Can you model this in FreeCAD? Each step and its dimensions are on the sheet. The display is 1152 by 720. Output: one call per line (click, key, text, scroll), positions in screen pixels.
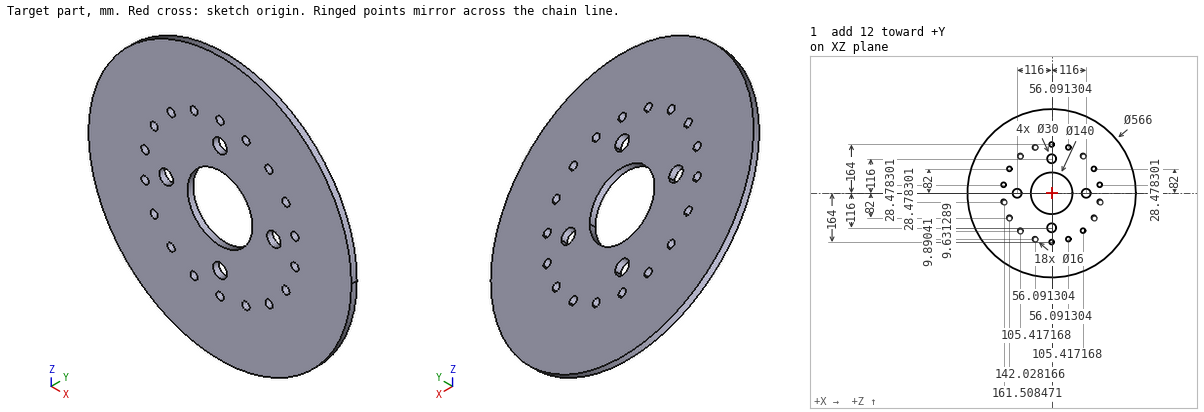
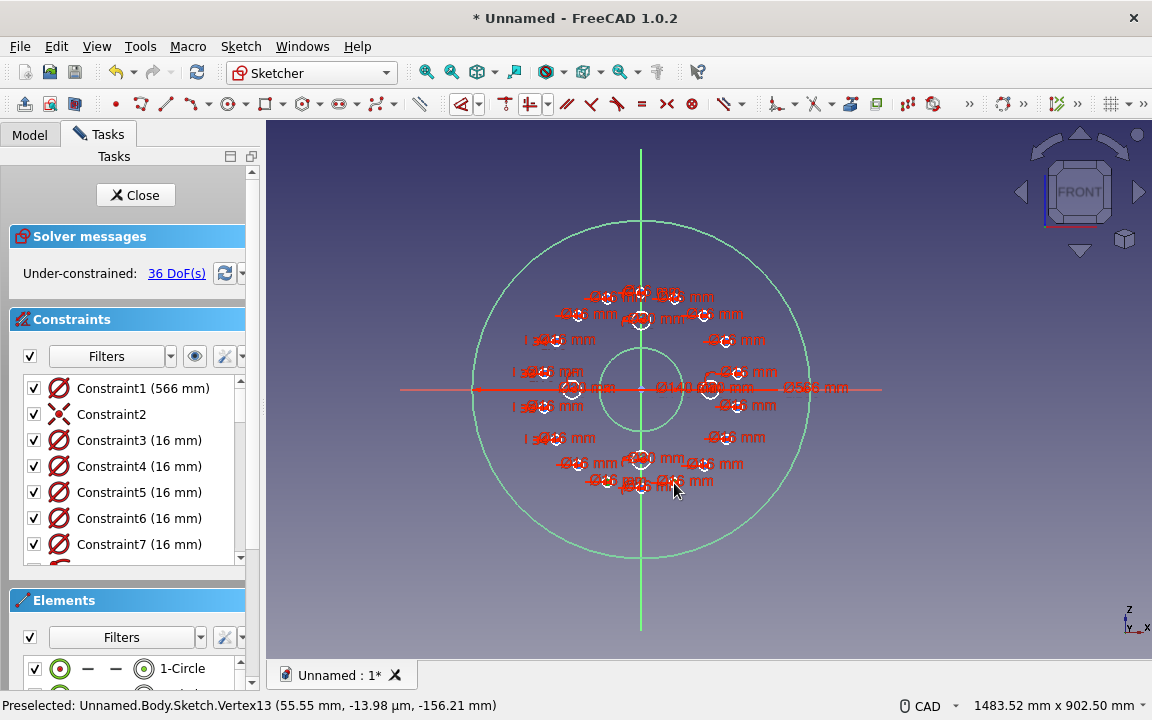
key(h)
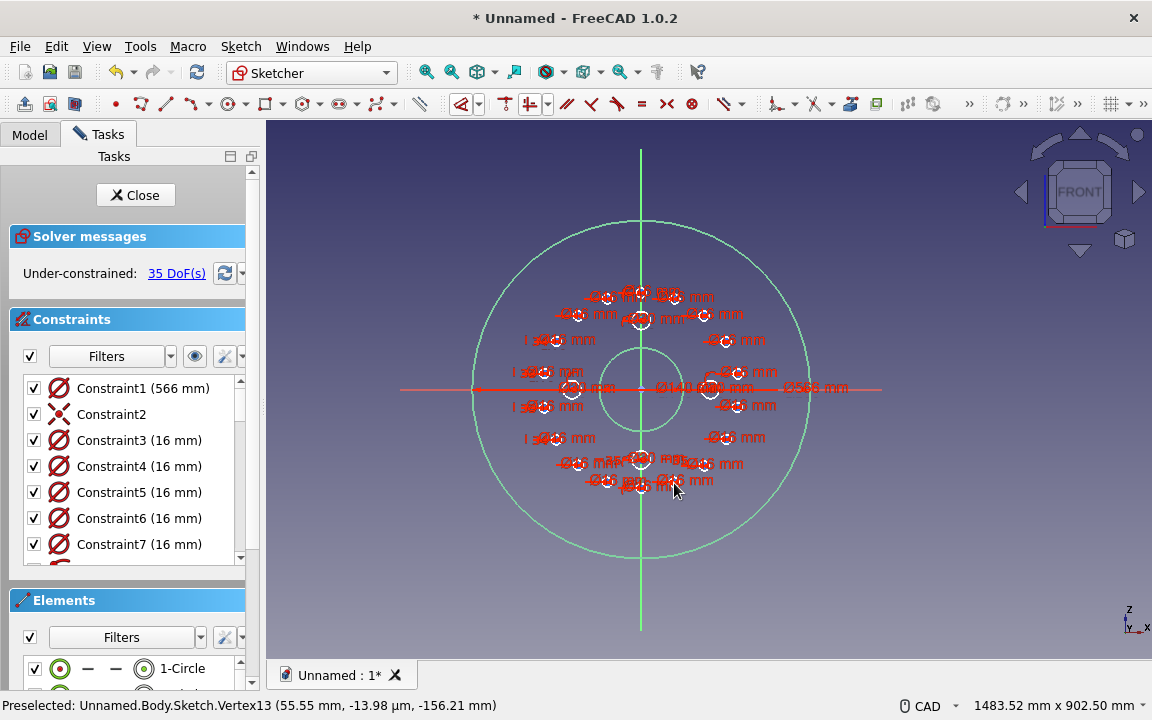
click(578, 465)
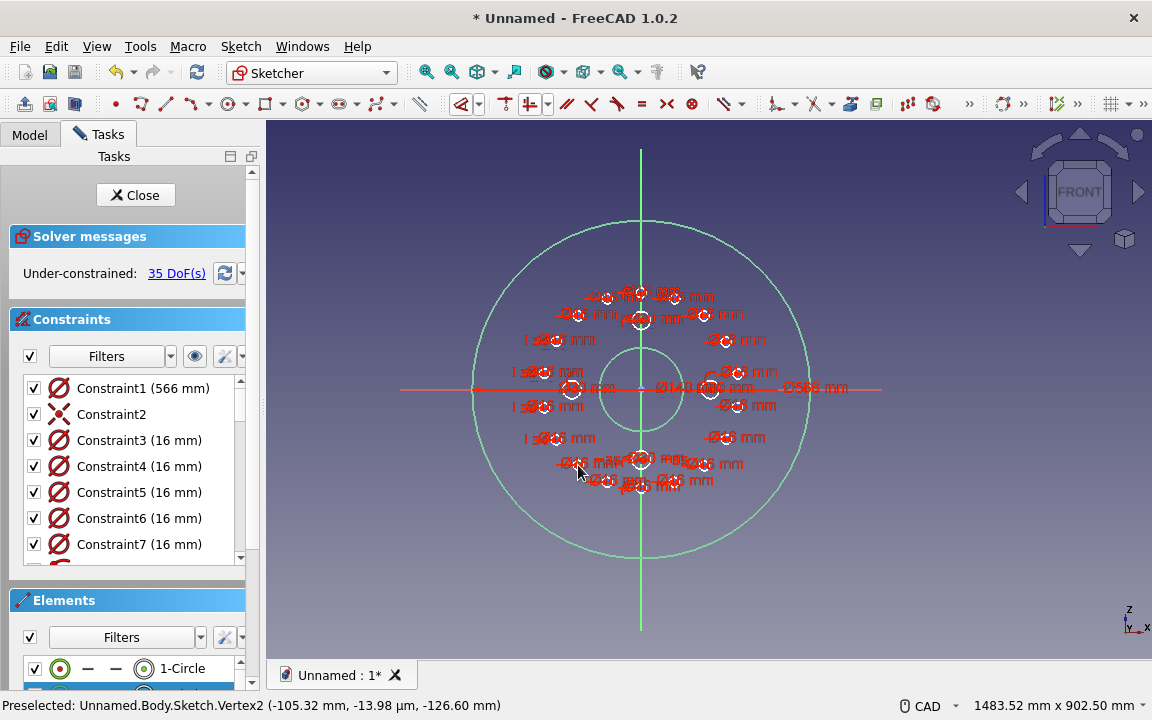
click(704, 466)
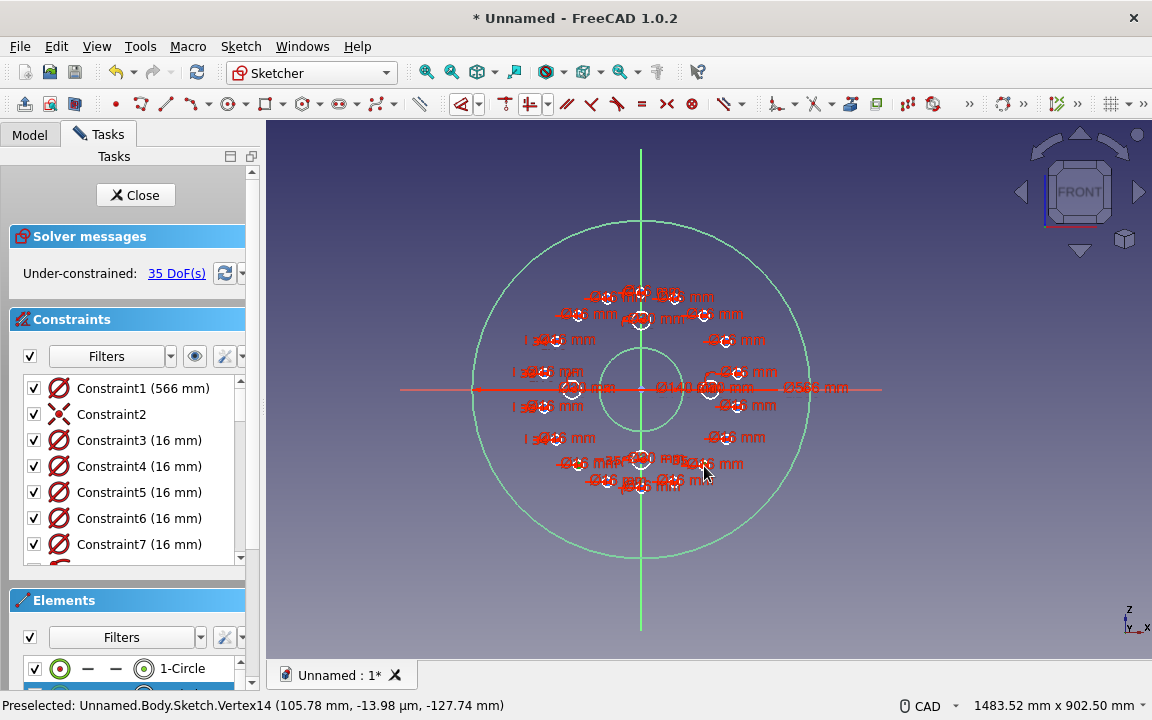
click(548, 104)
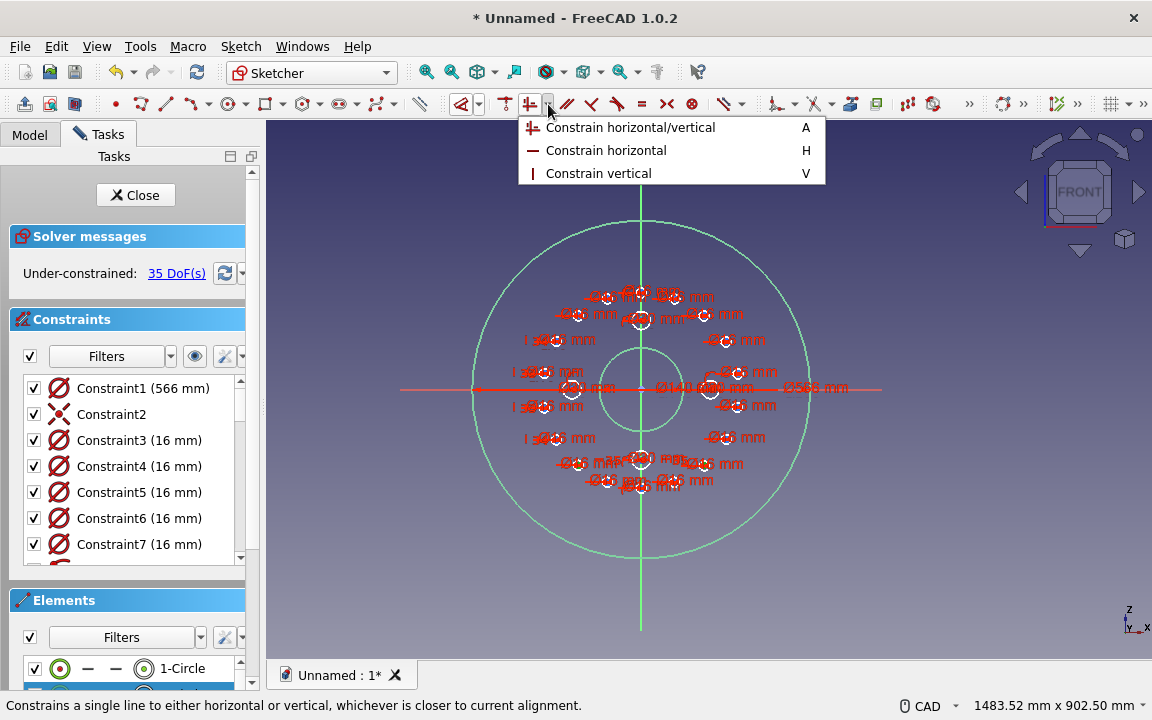
click(672, 150)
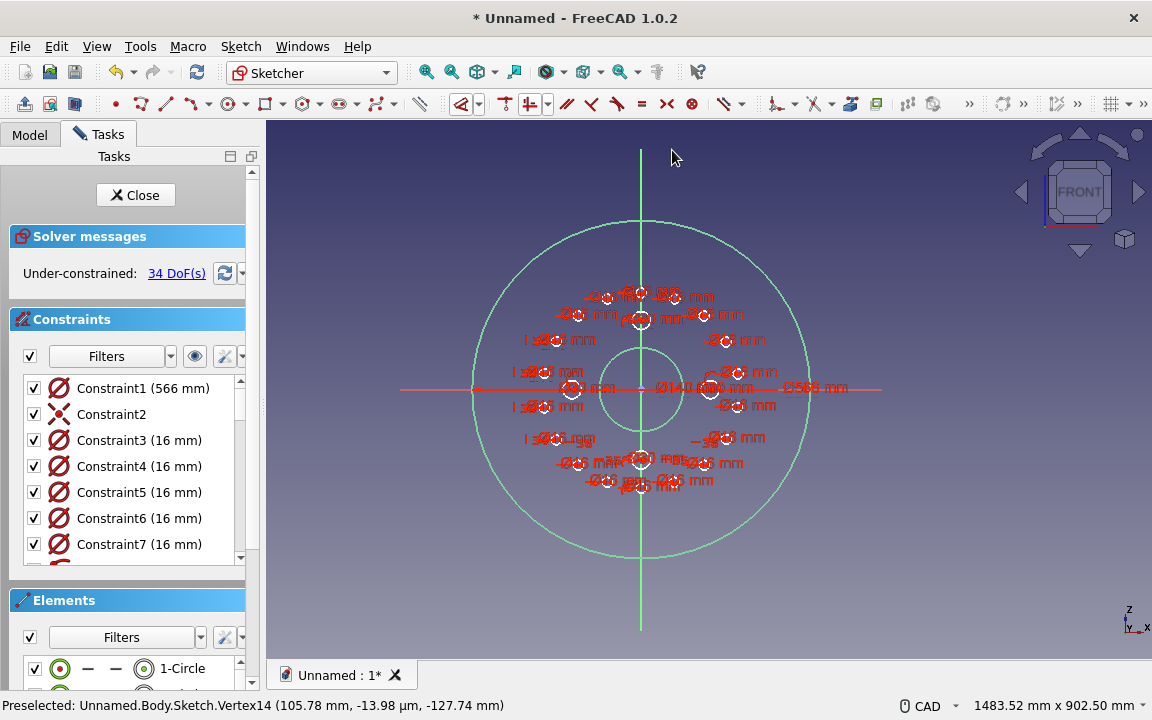
click(607, 299)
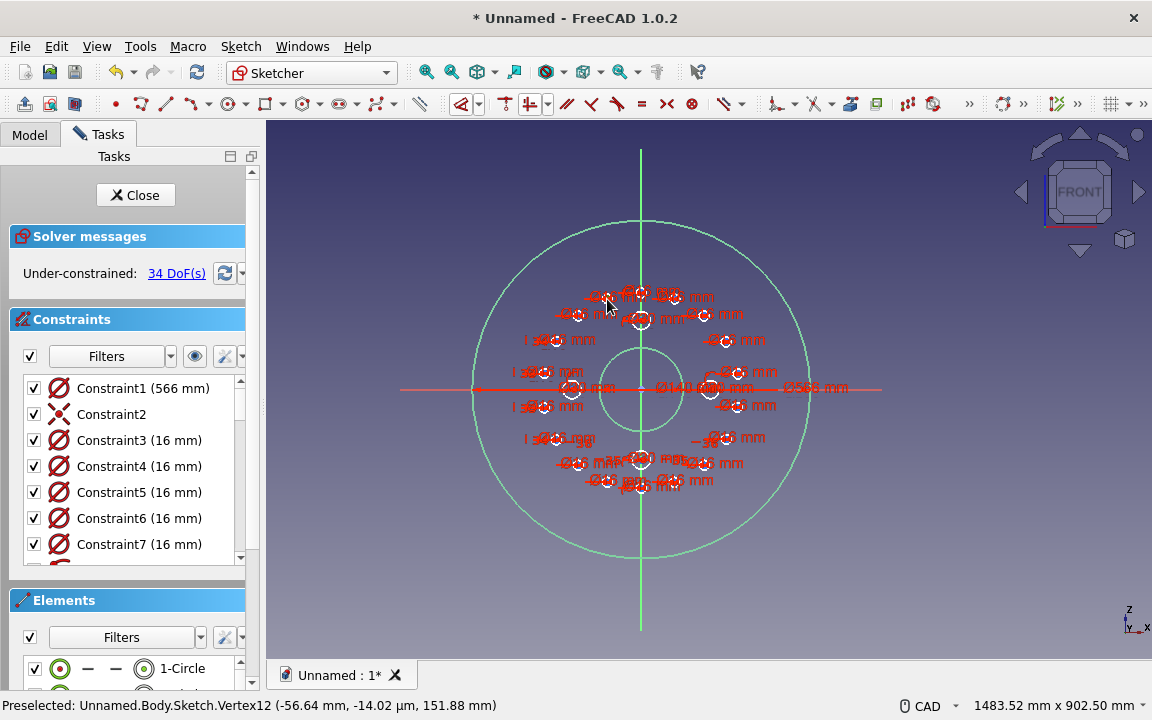
click(675, 299)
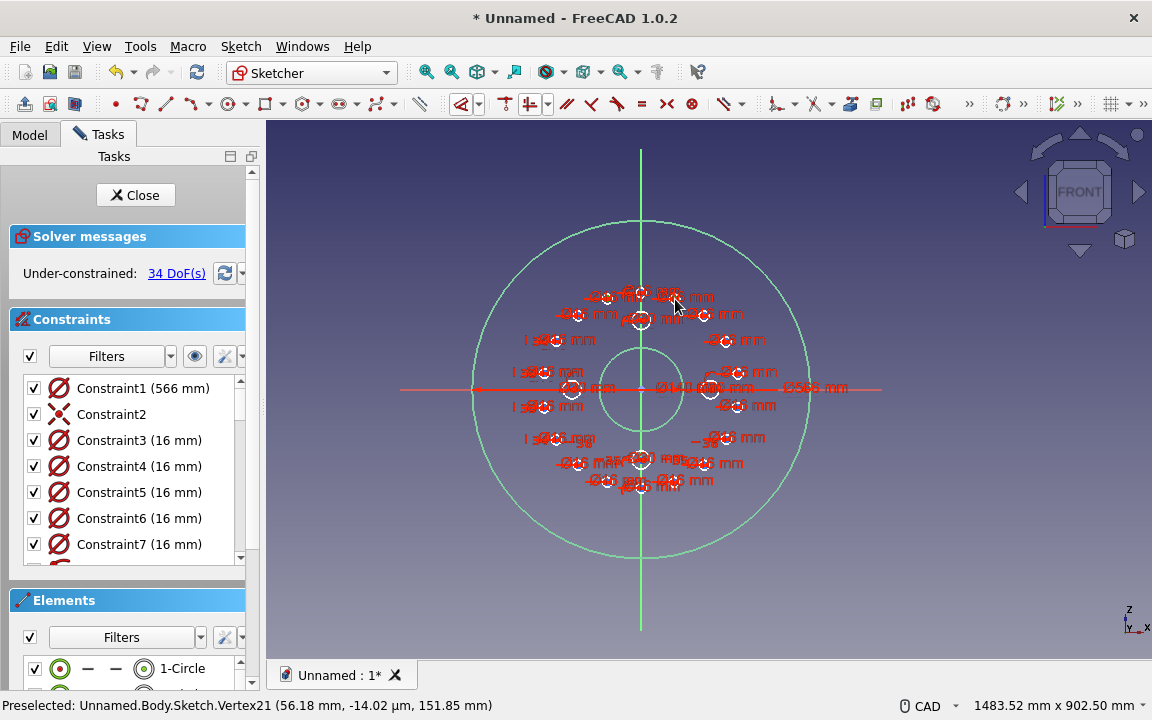
key(h)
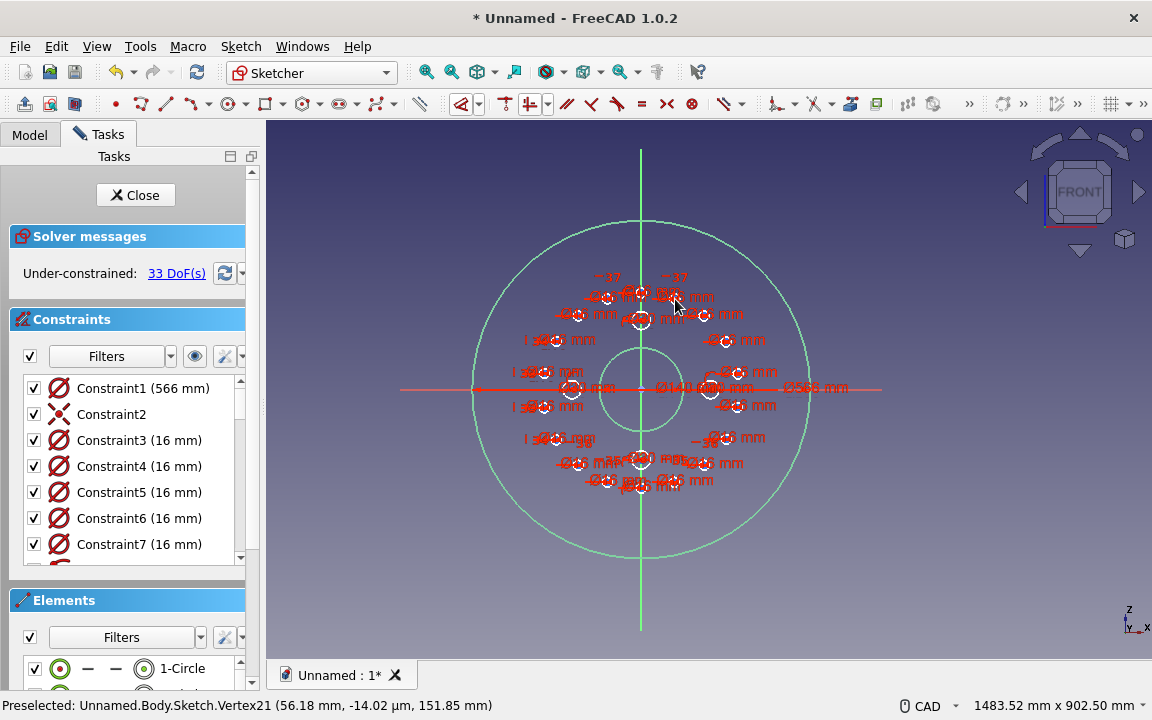
click(737, 407)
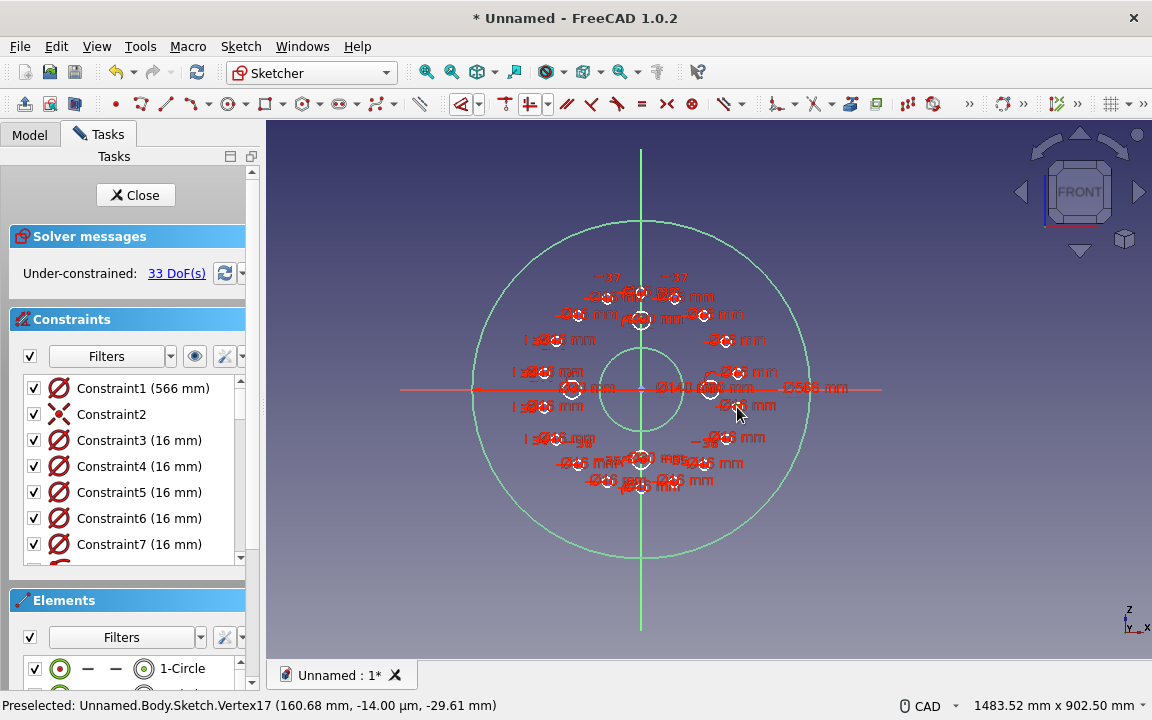
click(738, 374)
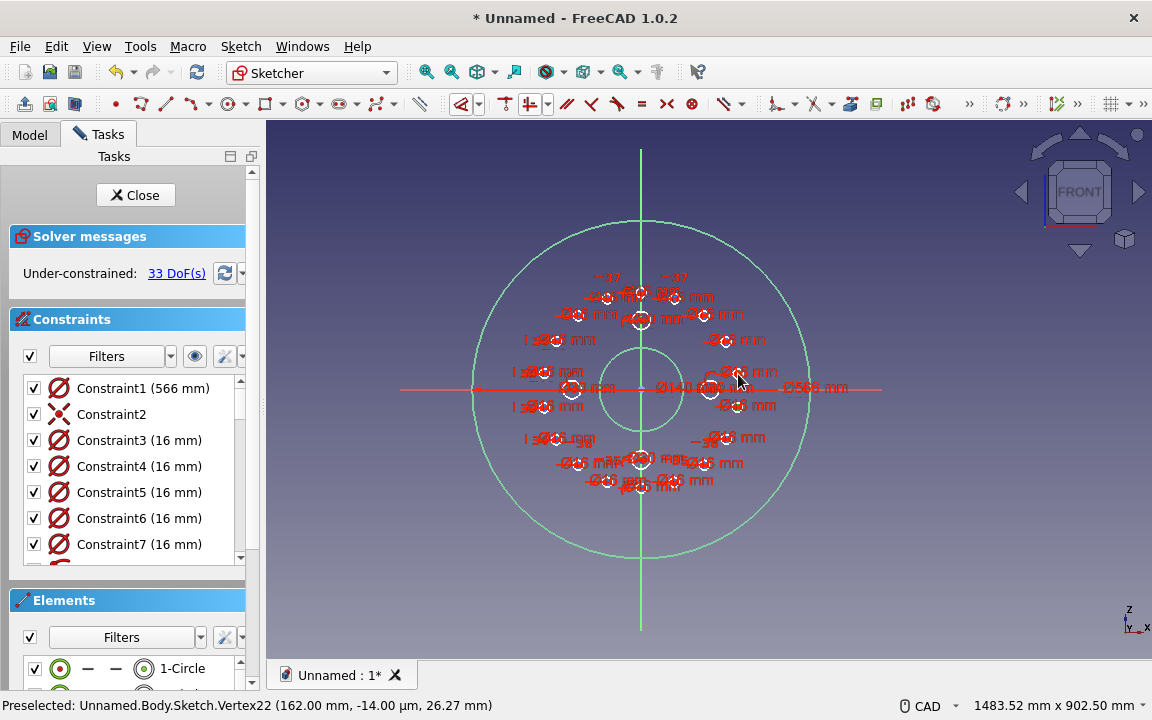
key(v)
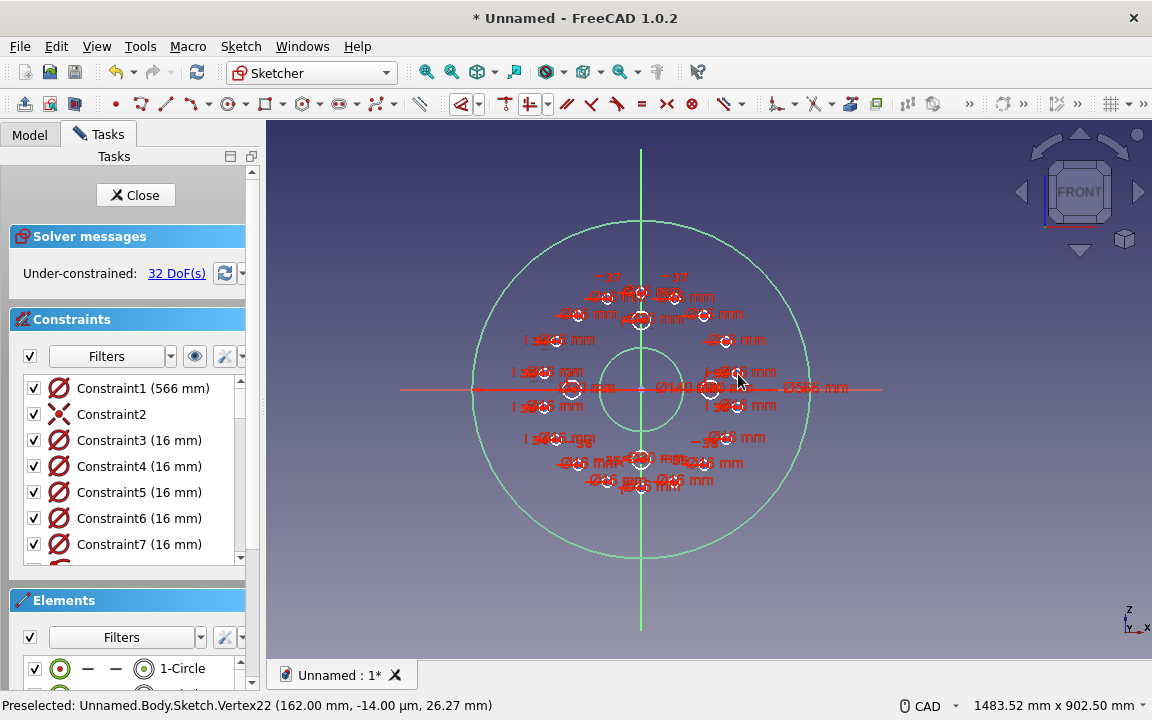
click(726, 439)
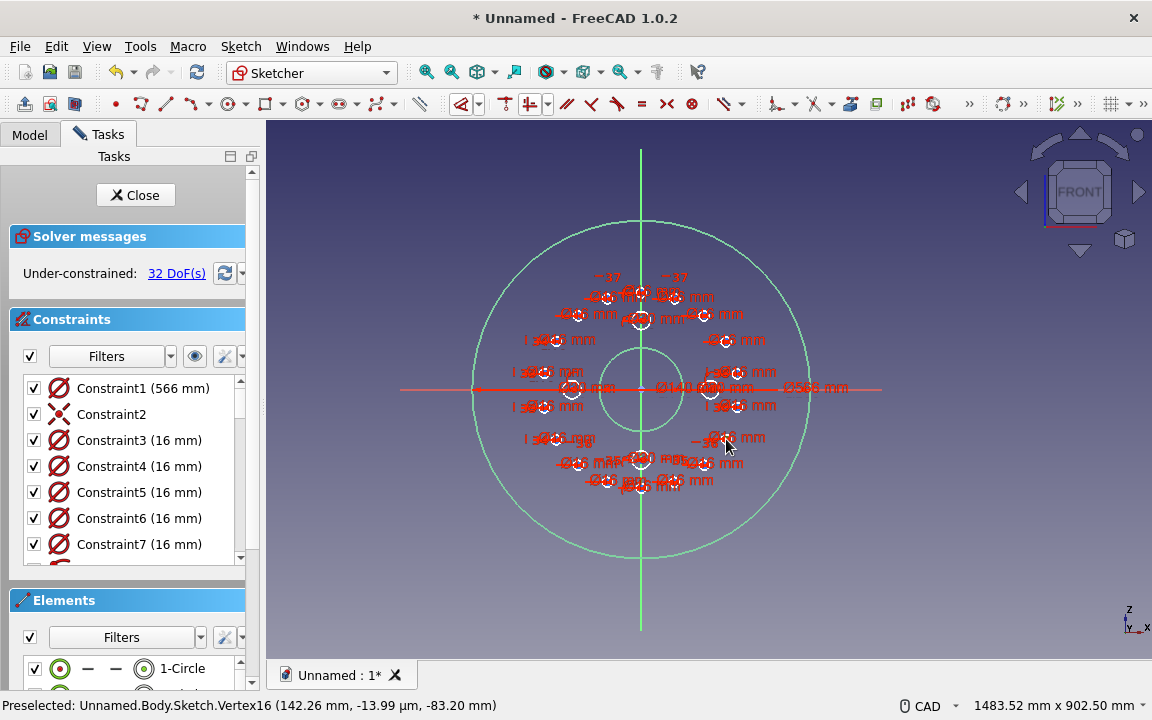
click(726, 342)